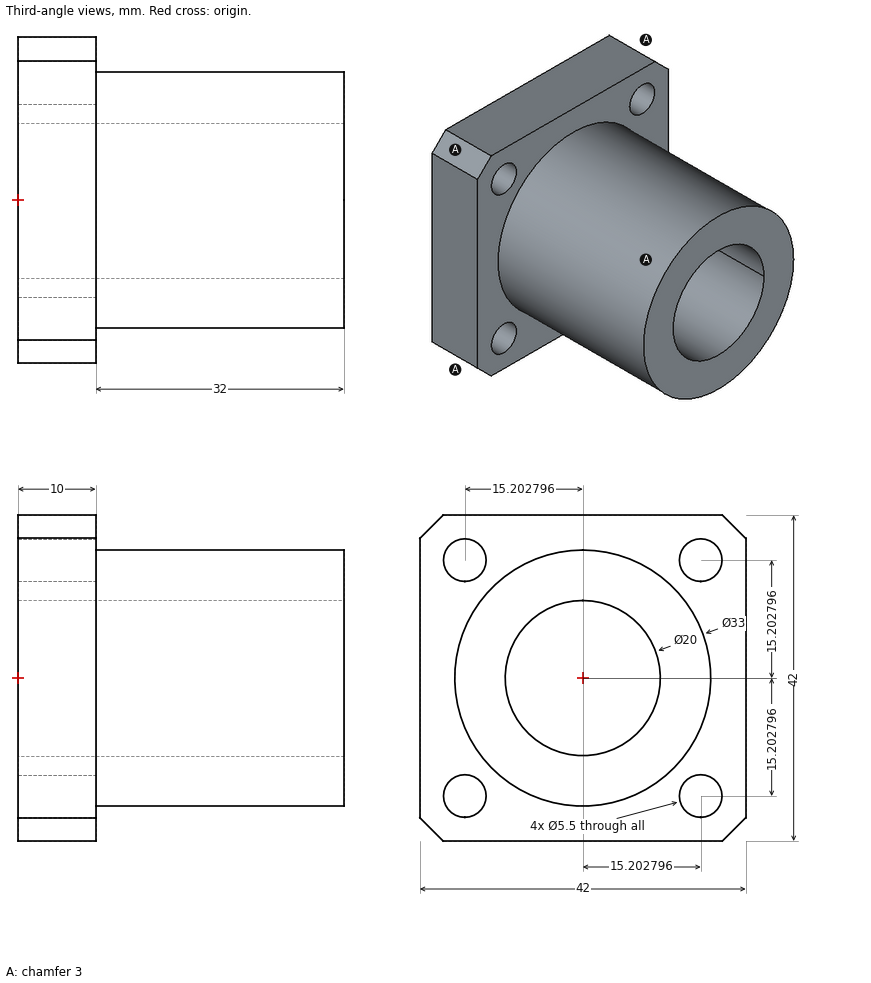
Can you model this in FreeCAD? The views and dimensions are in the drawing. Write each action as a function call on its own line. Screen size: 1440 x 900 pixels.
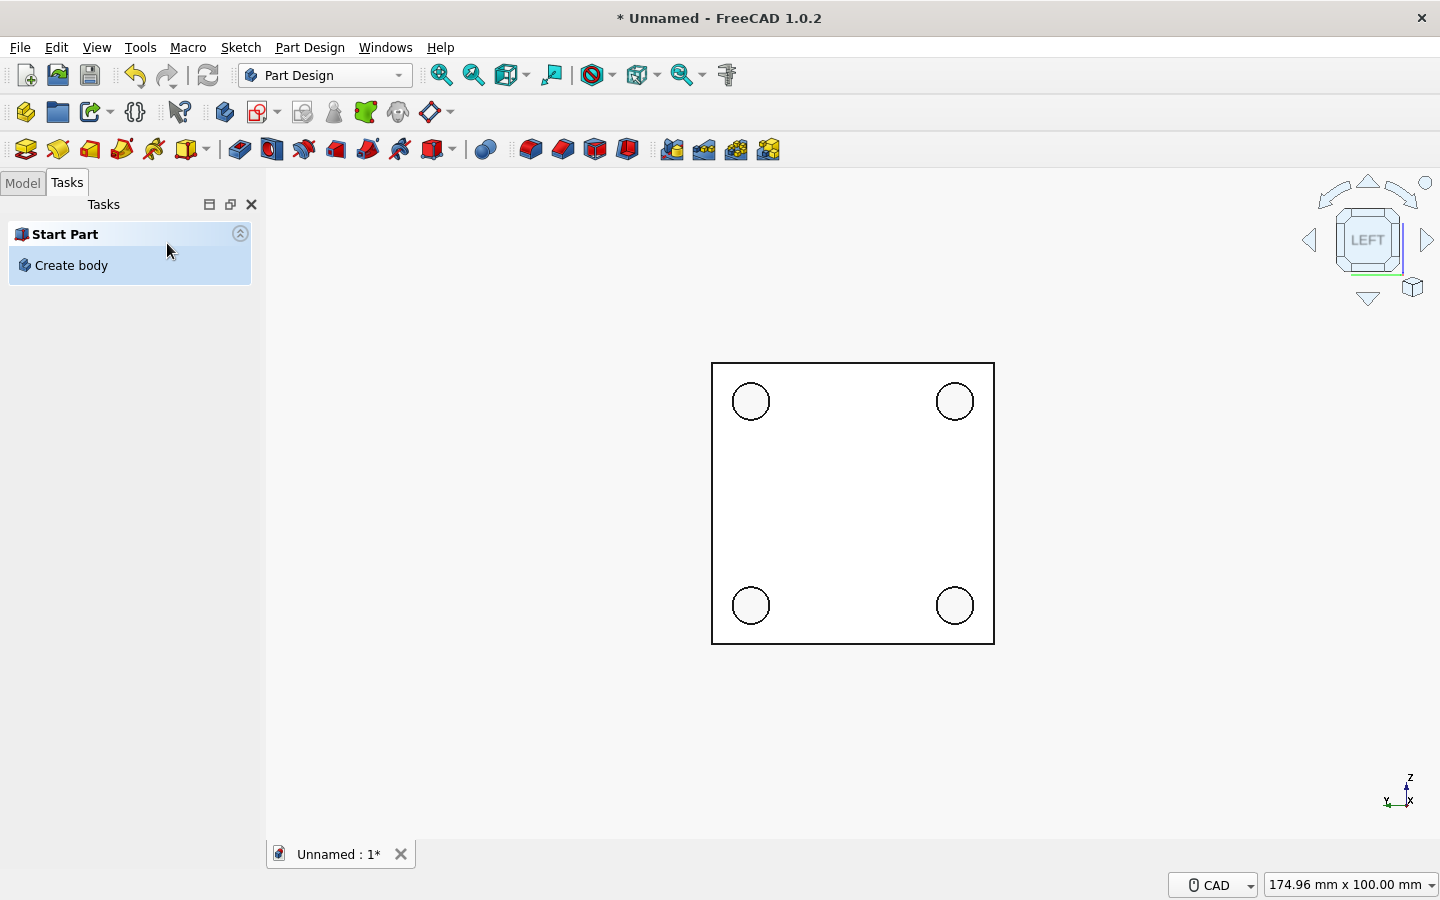
click(442, 76)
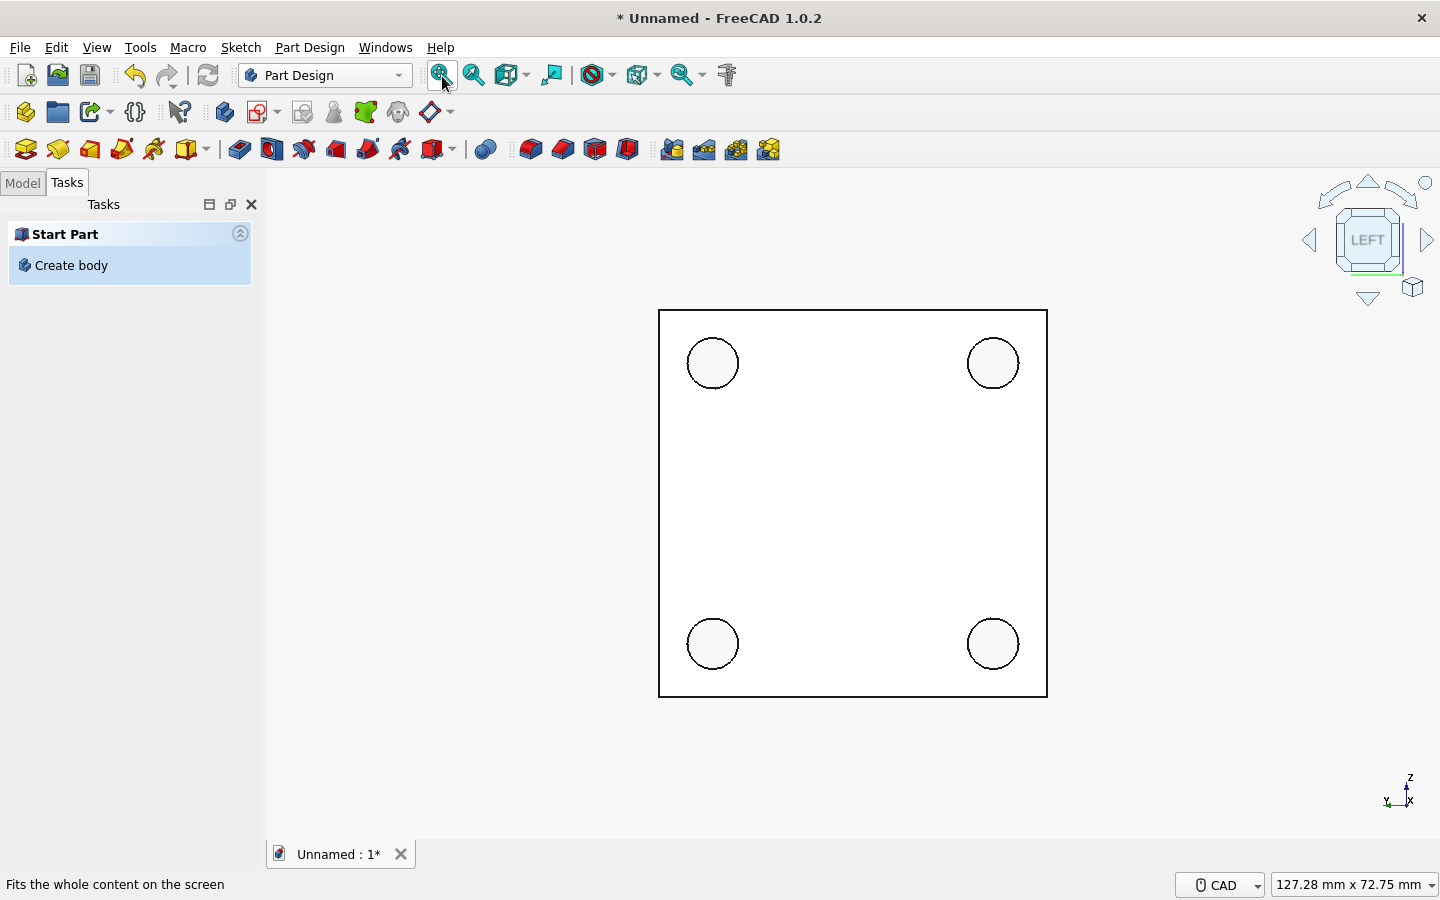
click(853, 502)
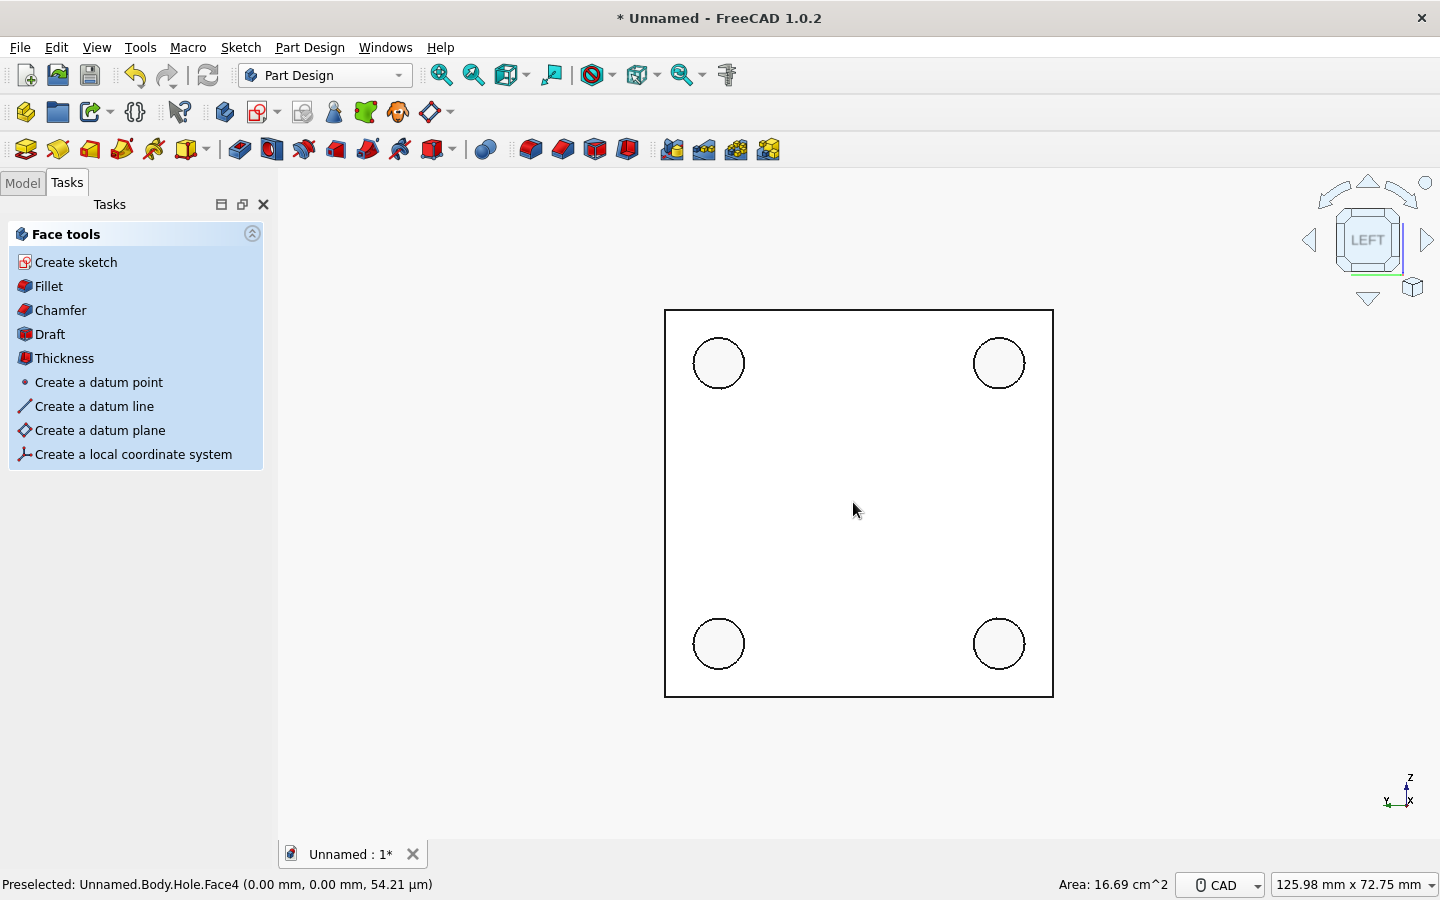
click(258, 112)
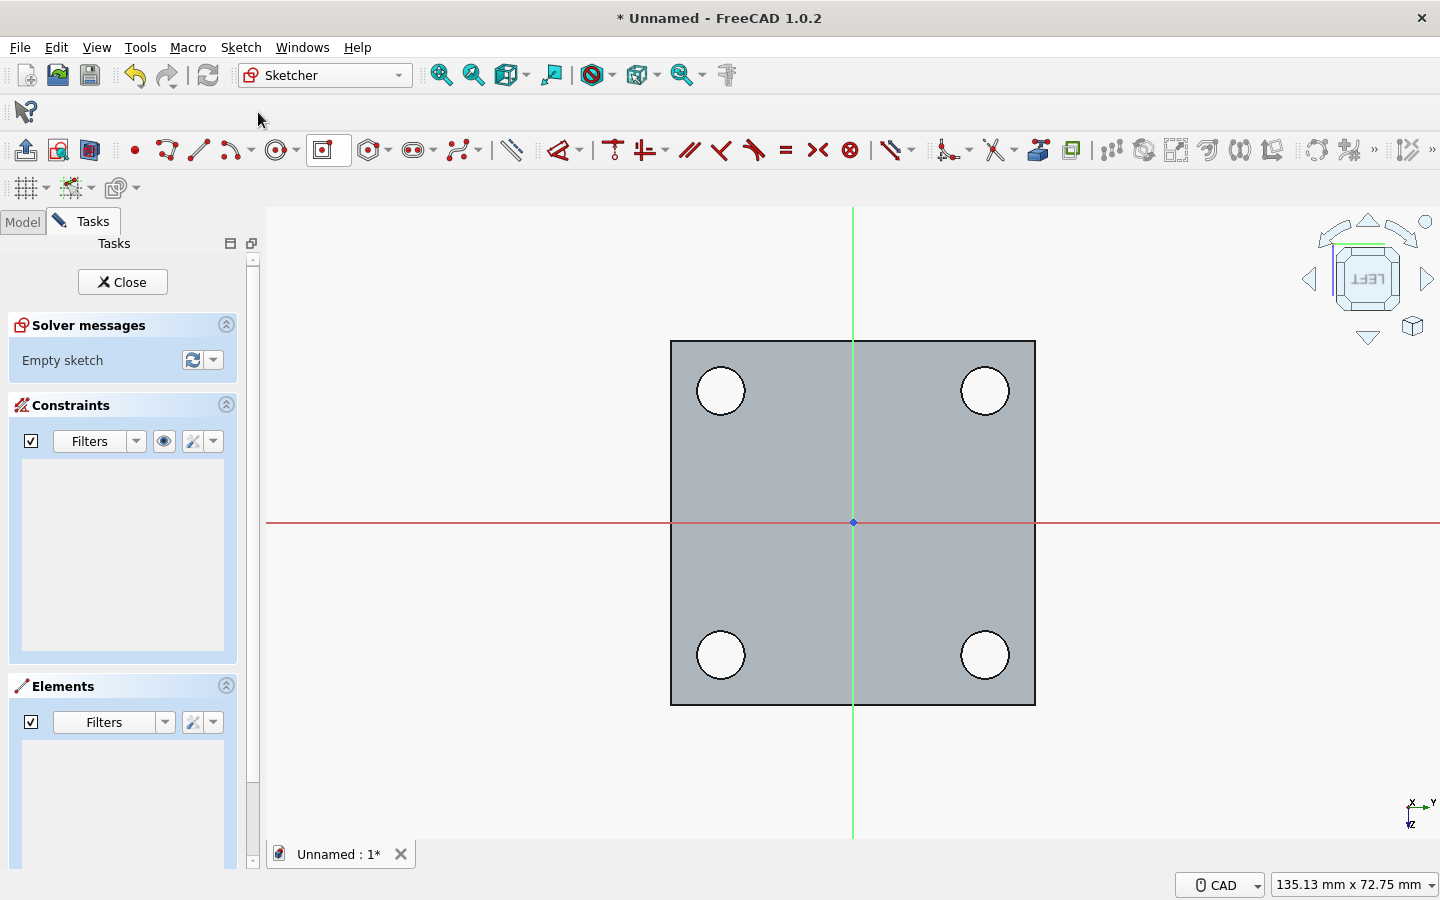
scroll(909, 523, up, 4)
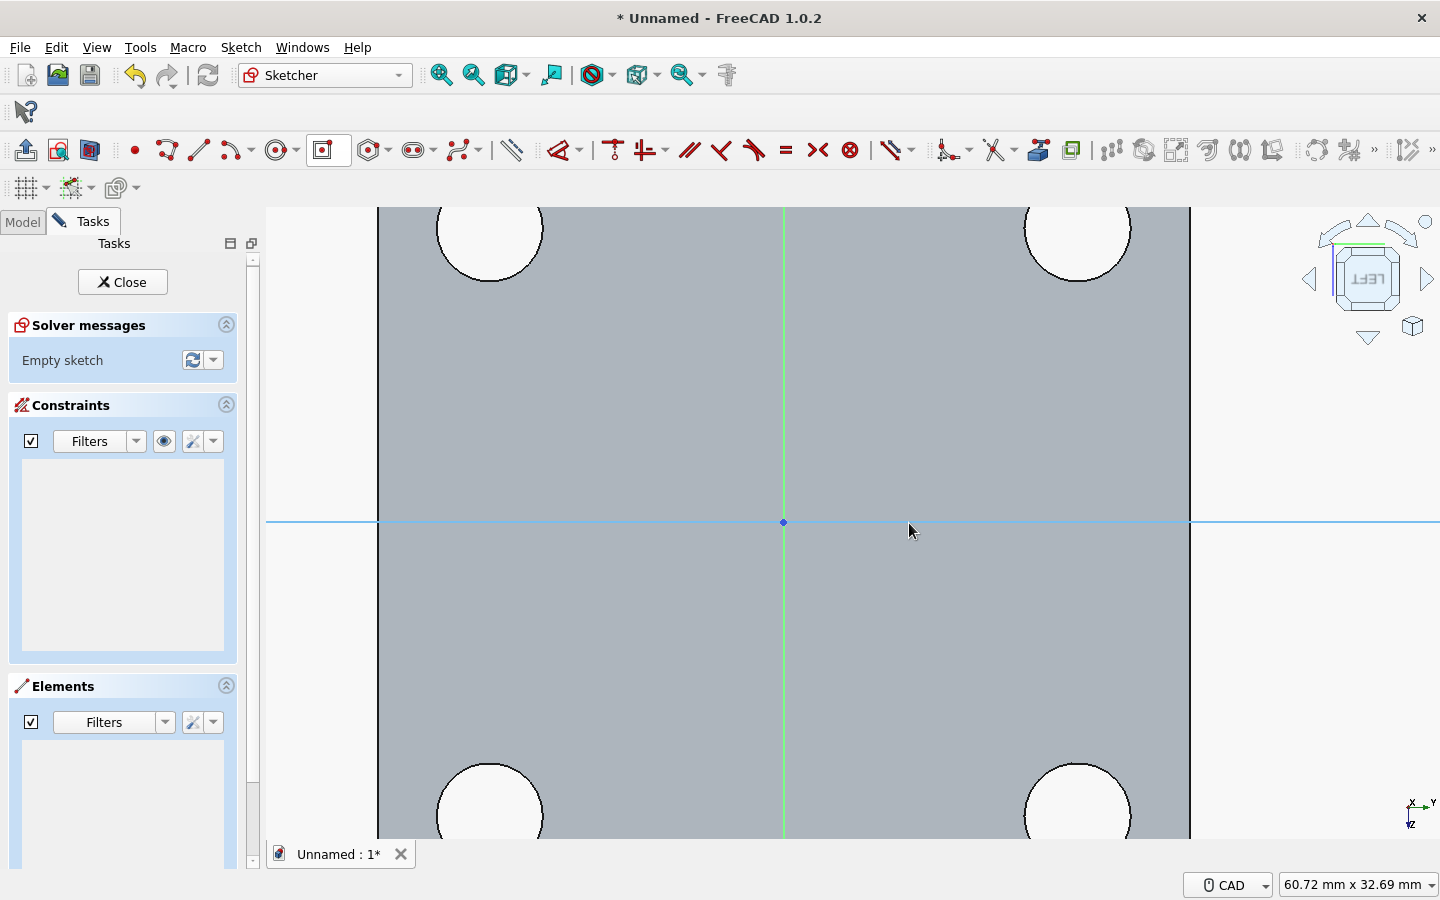
click(276, 150)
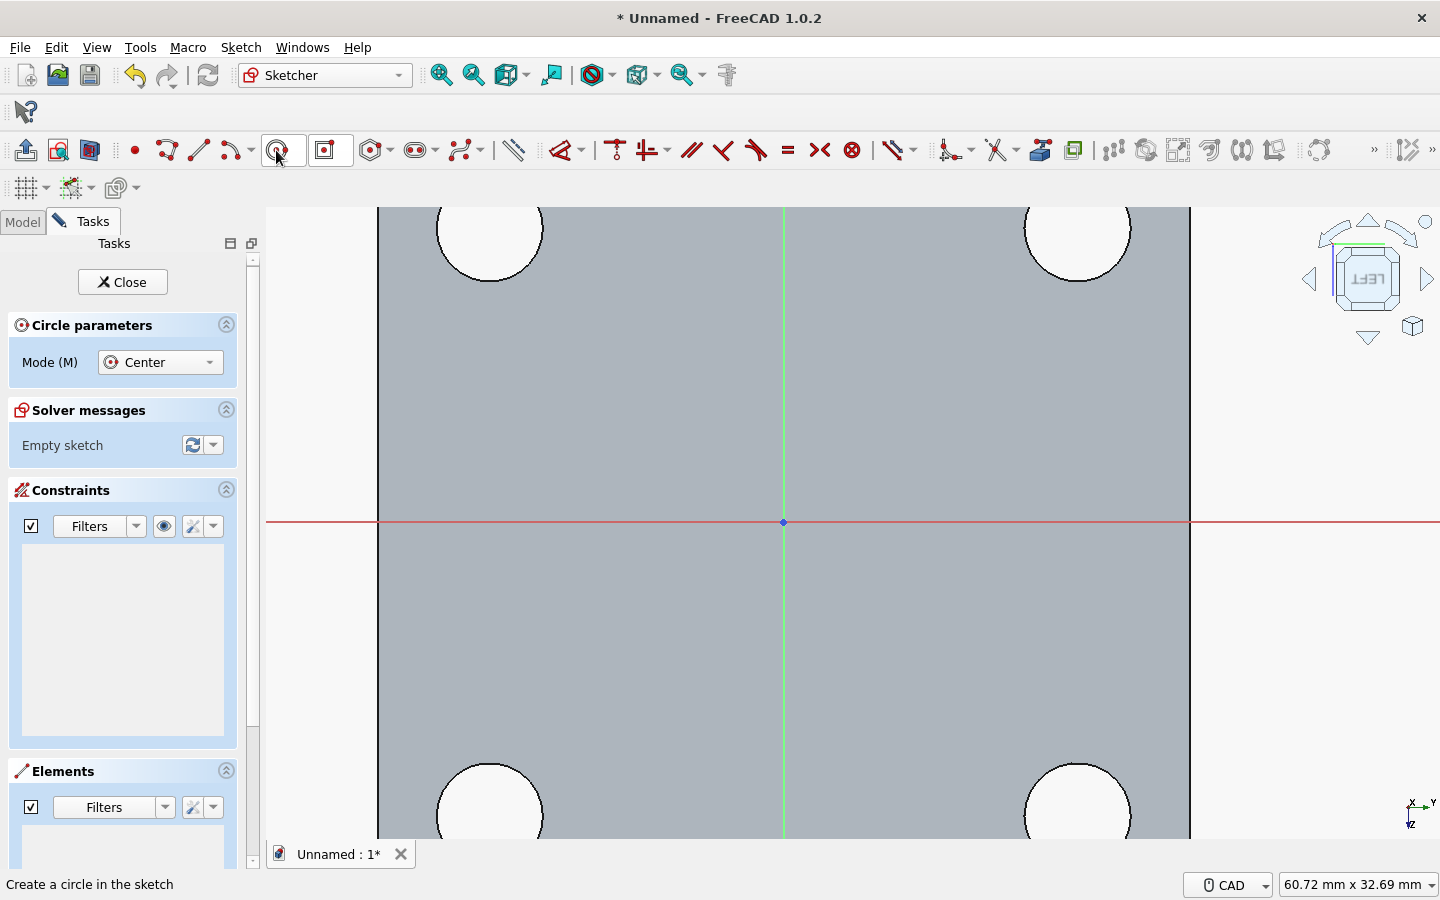
click(784, 522)
click(920, 386)
key(Escape)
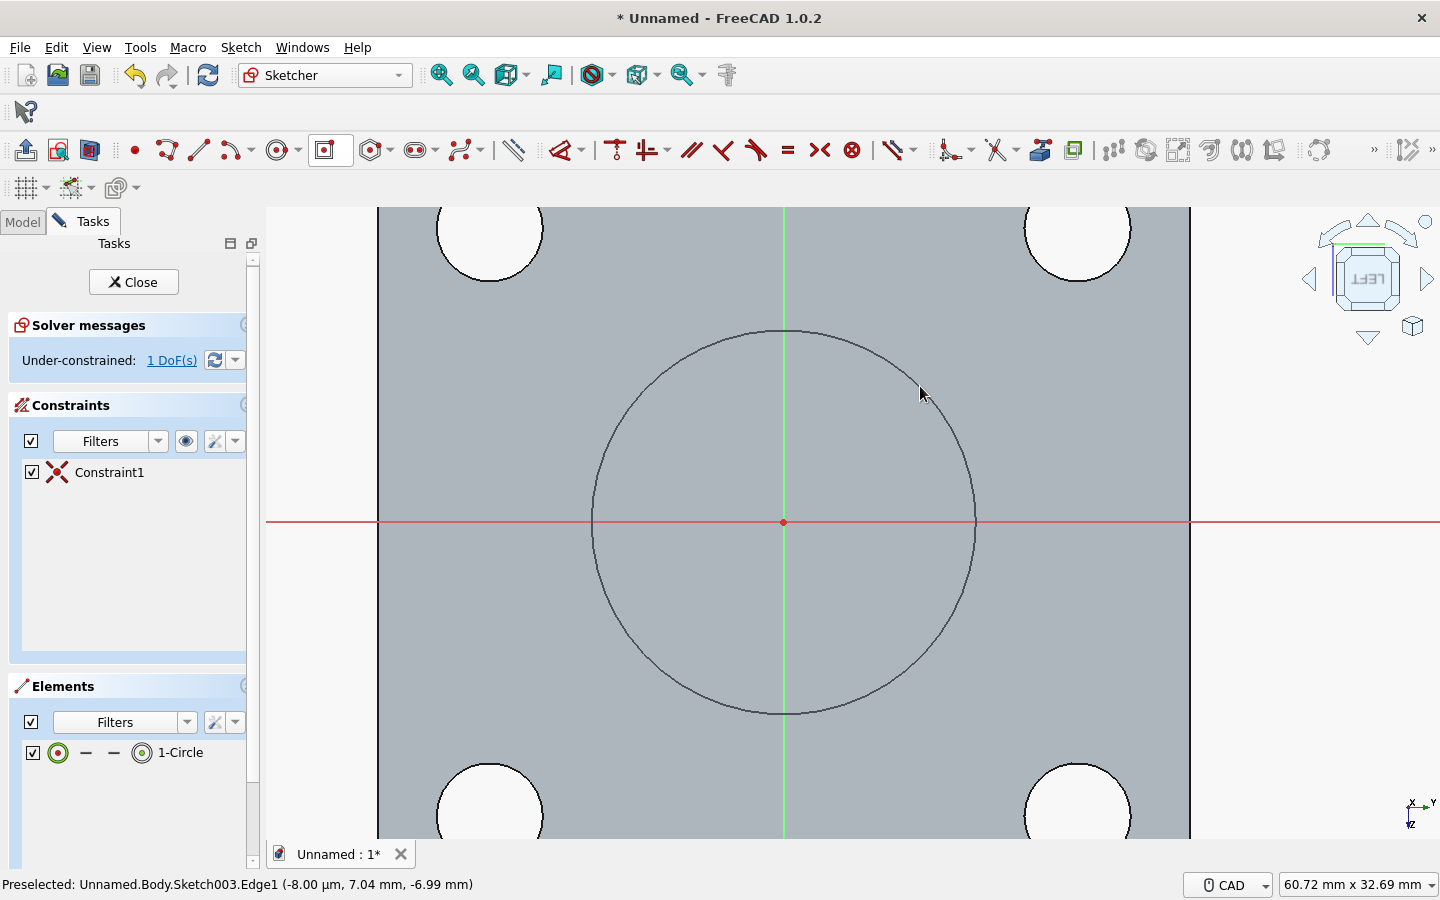
click(560, 150)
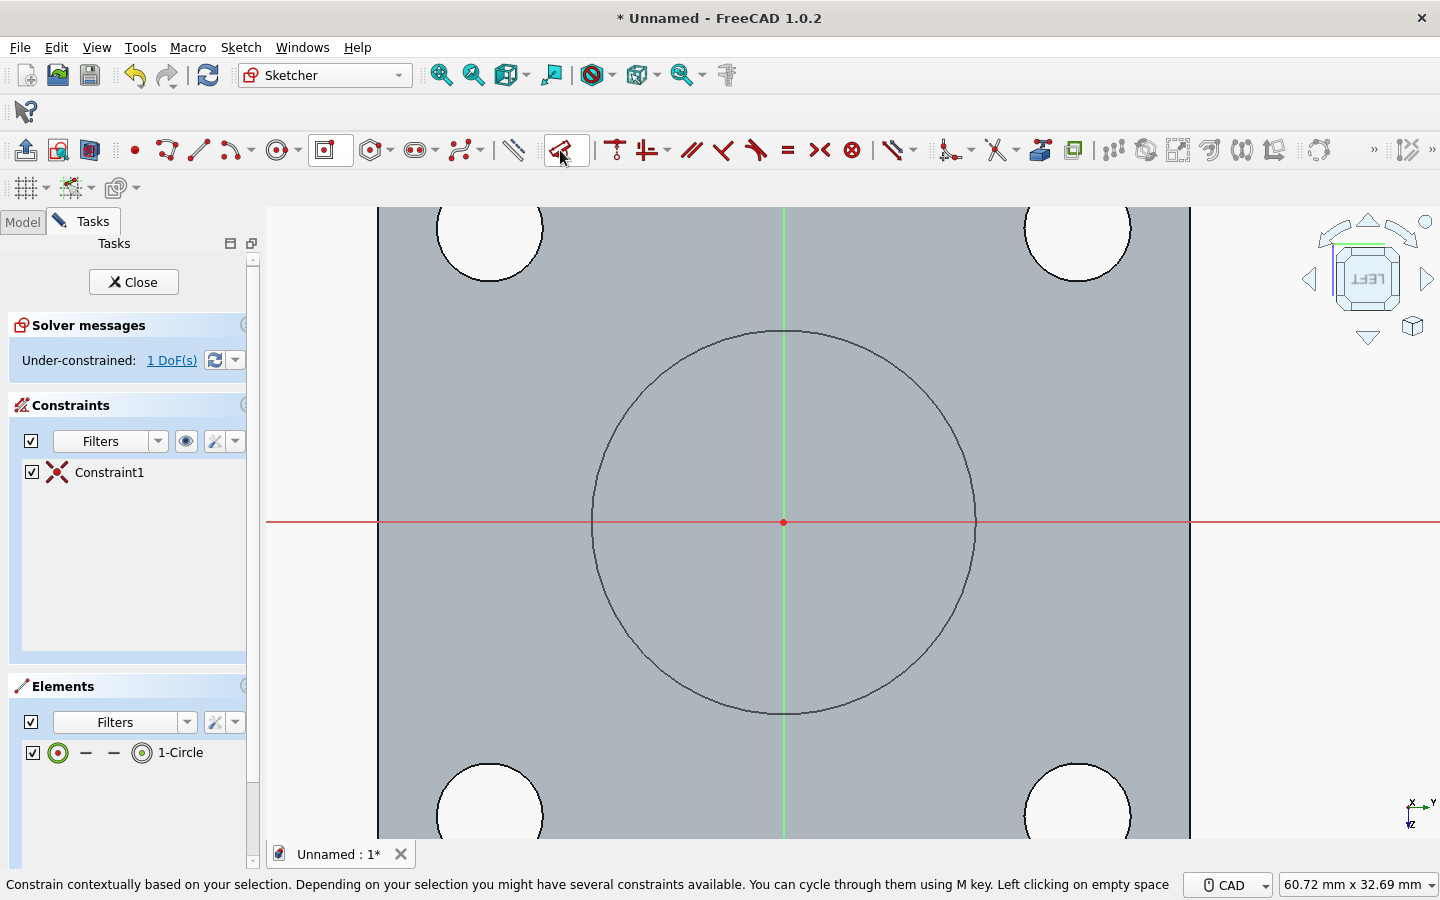
click(919, 386)
click(942, 363)